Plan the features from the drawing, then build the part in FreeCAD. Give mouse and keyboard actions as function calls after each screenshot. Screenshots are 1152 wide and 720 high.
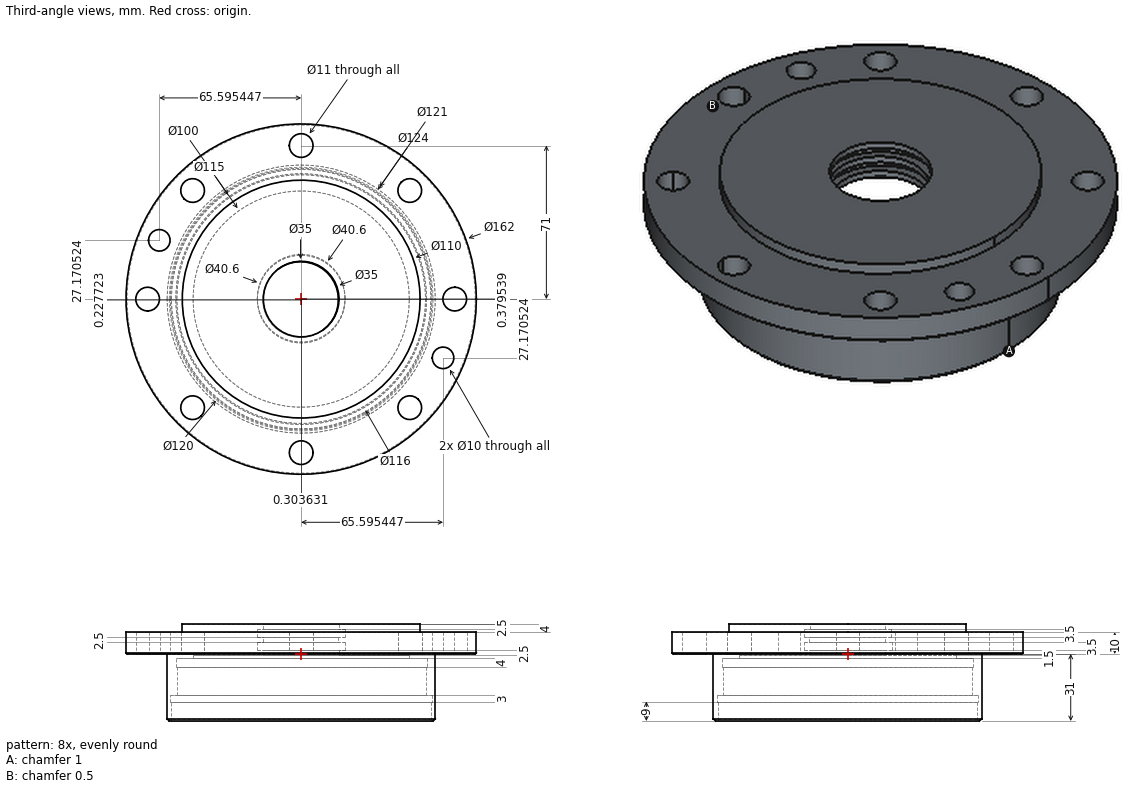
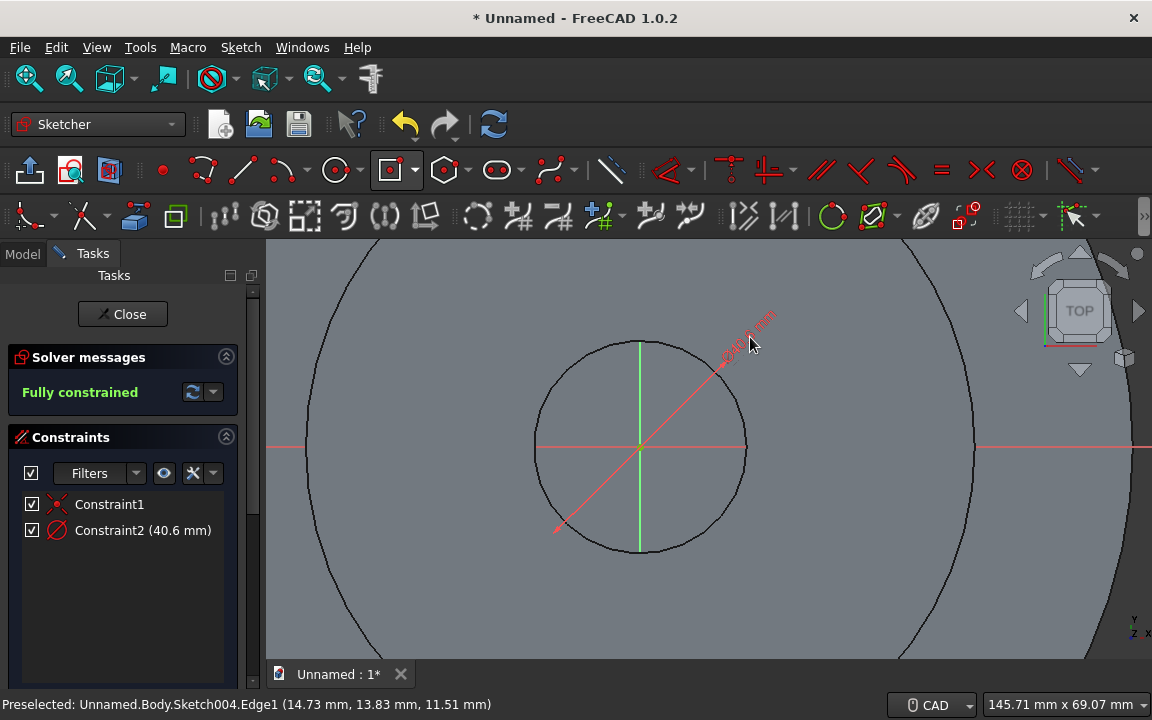
click(123, 314)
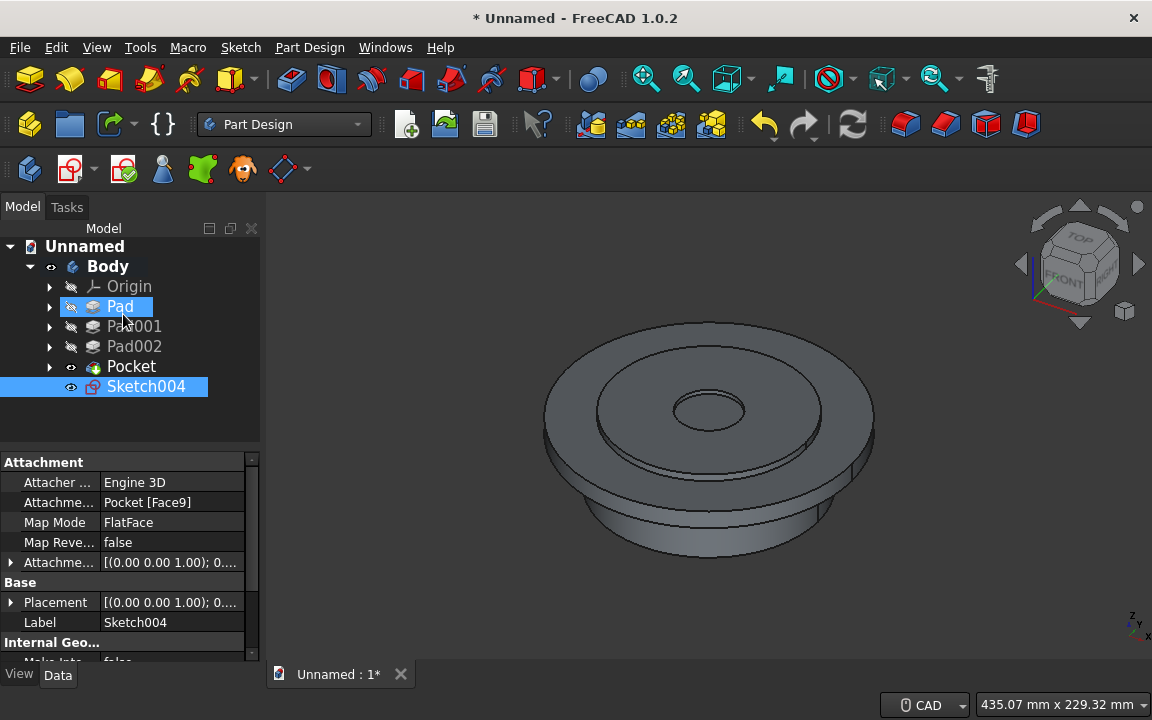
click(292, 80)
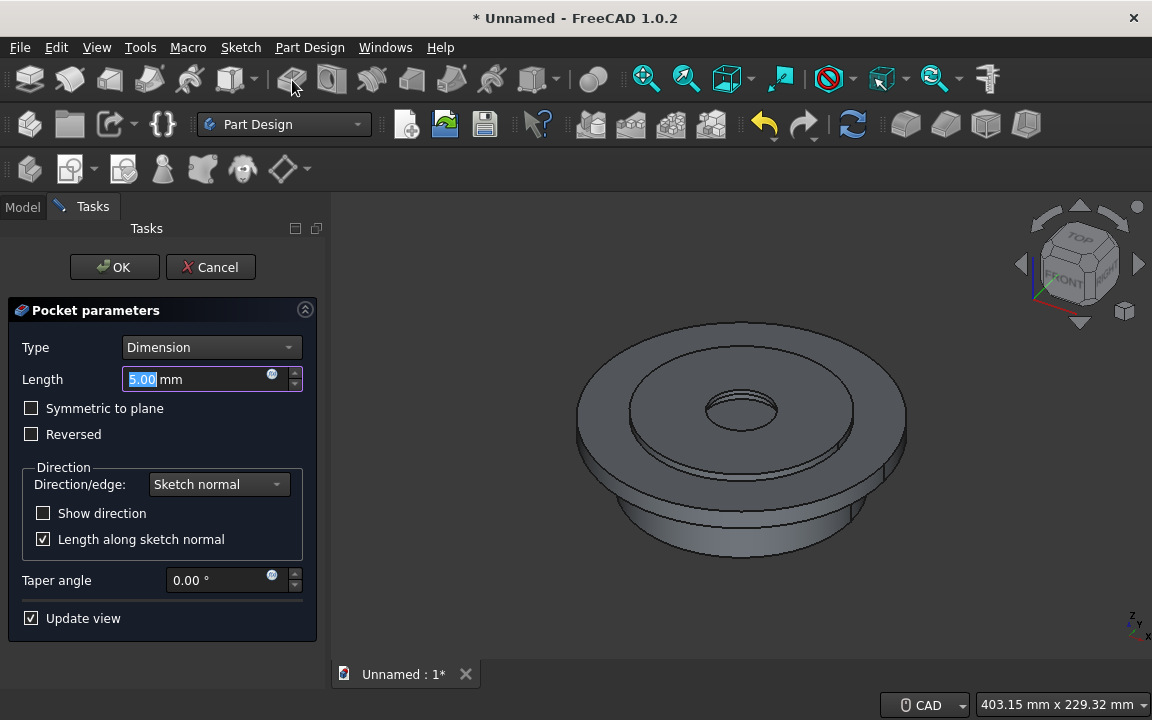
text(3.5)
key(Tab)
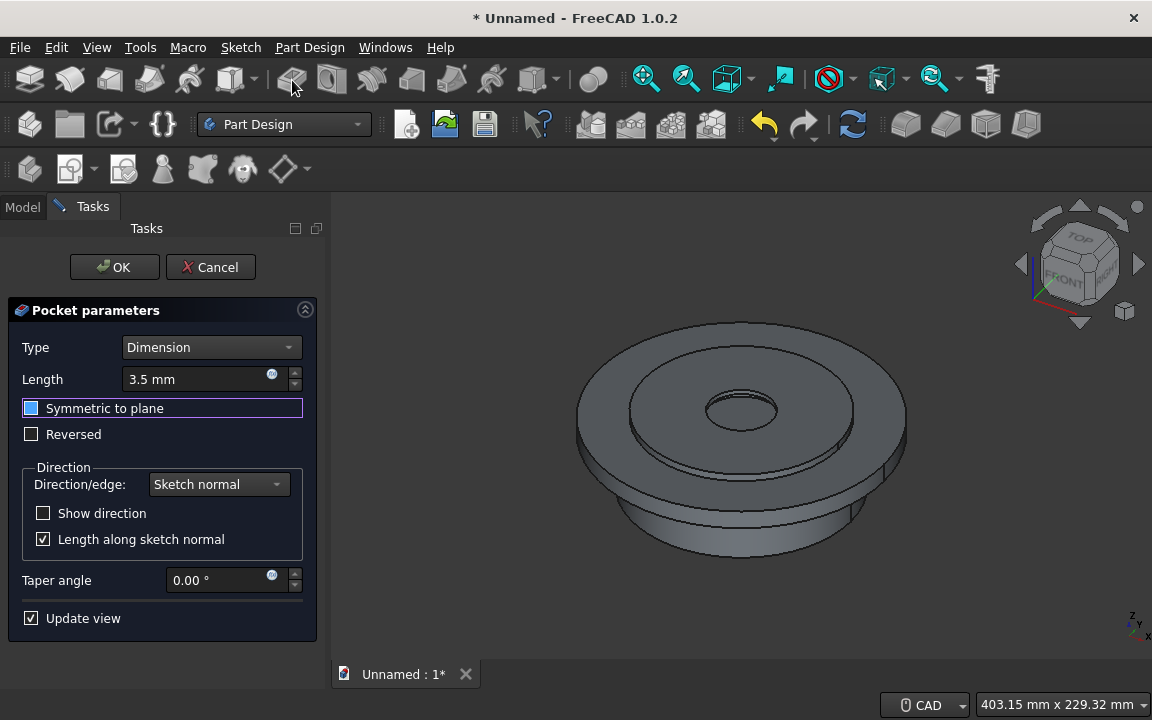
click(115, 267)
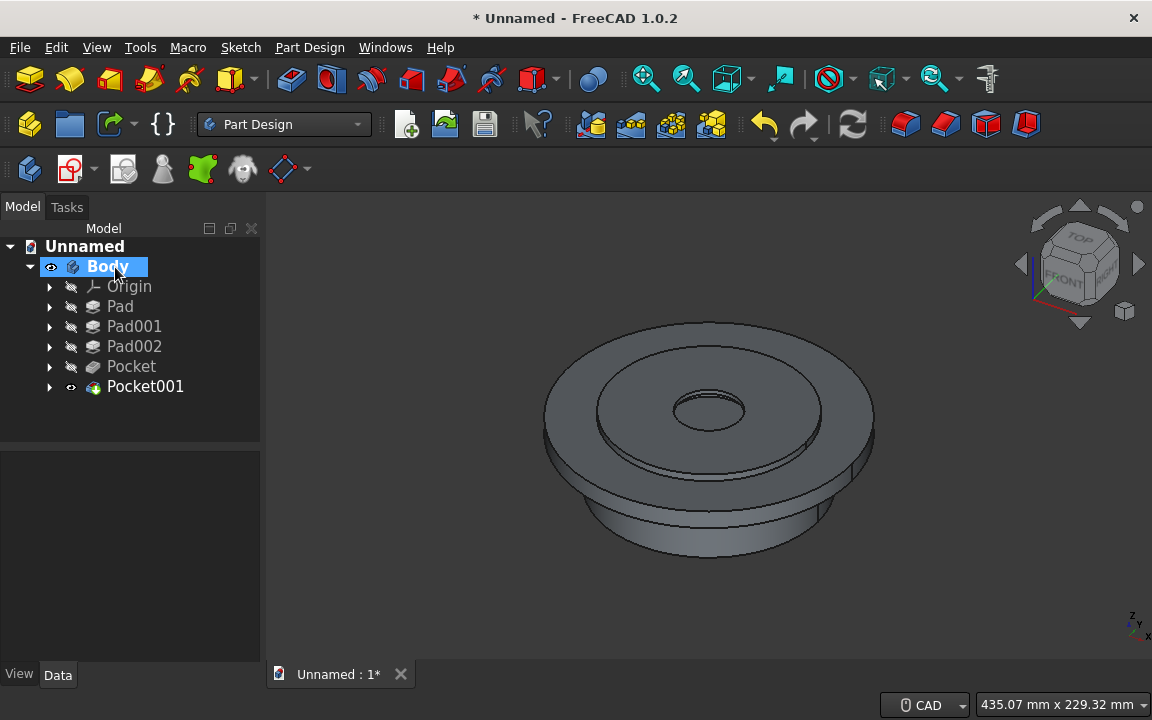
click(709, 419)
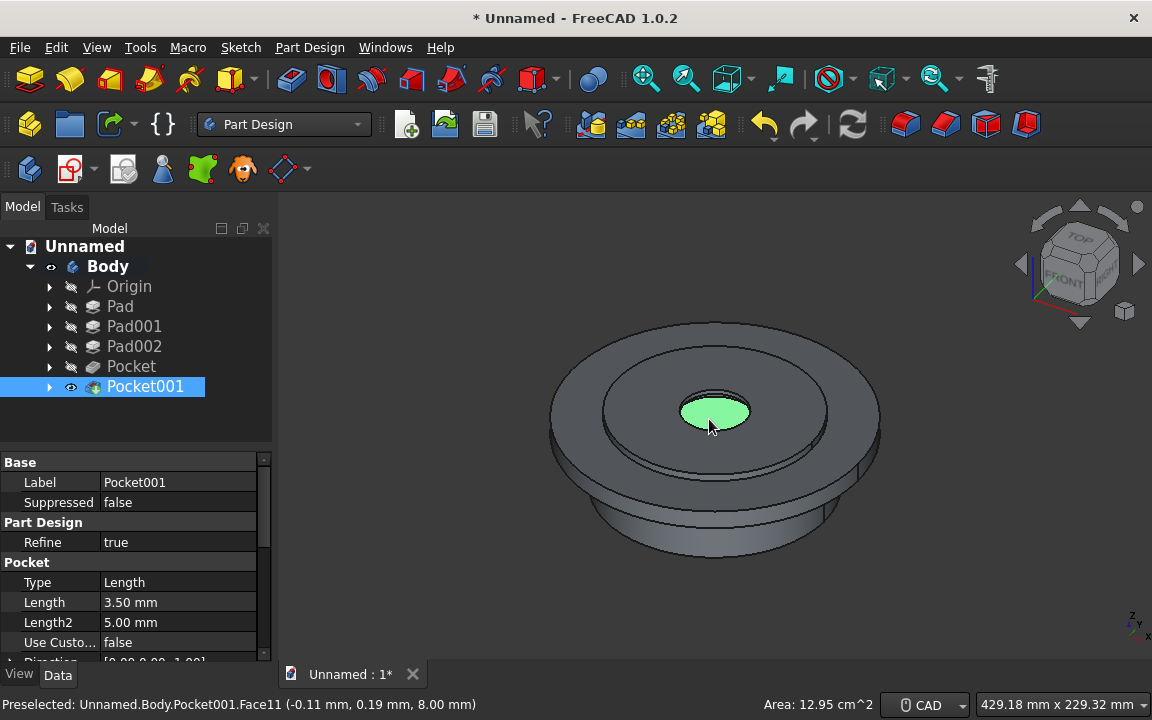
click(70, 170)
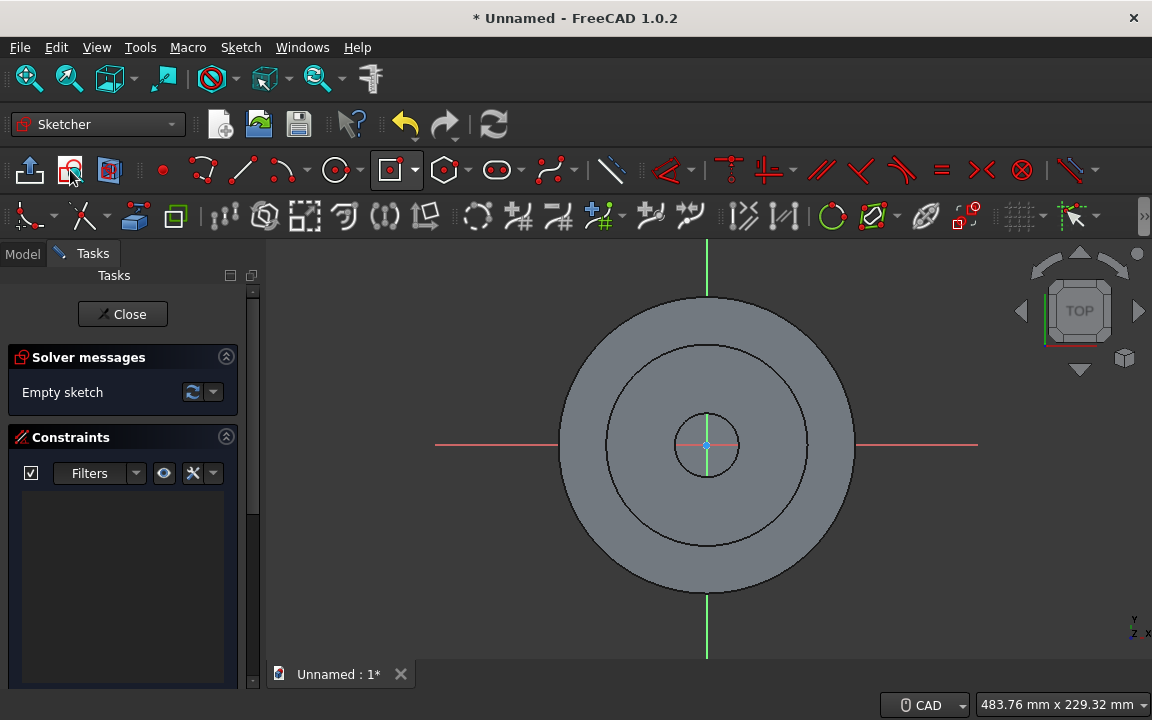
key(q)
key(s)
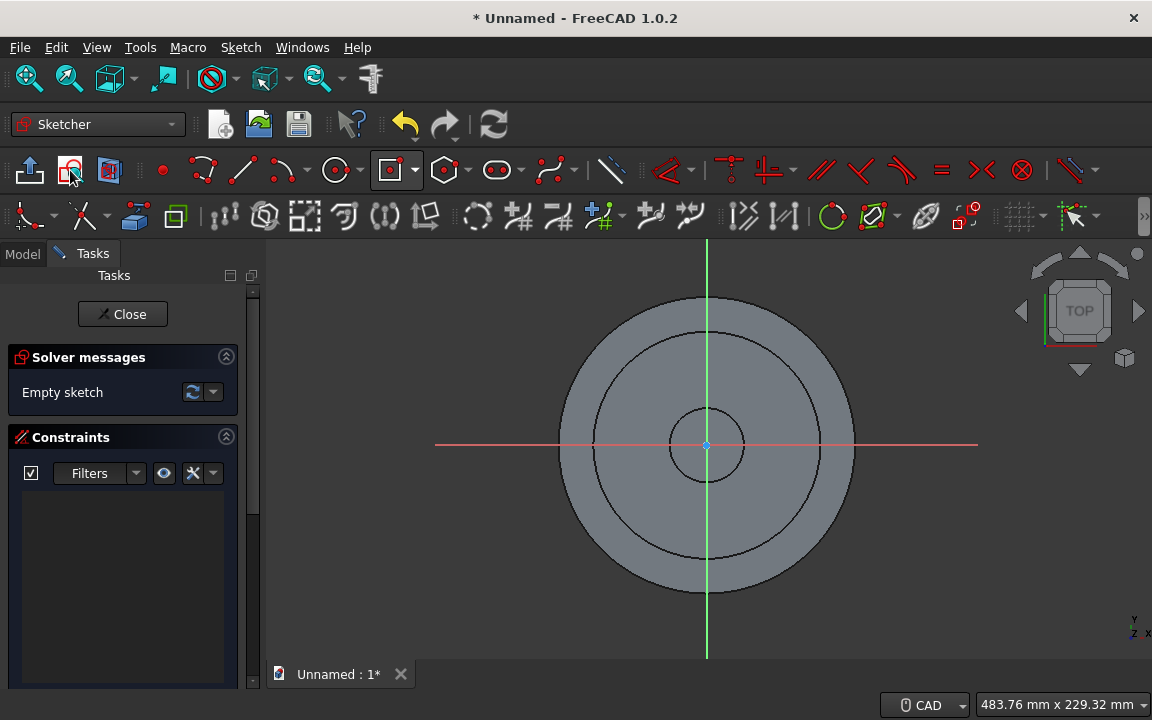
scroll(728, 445, up, 7)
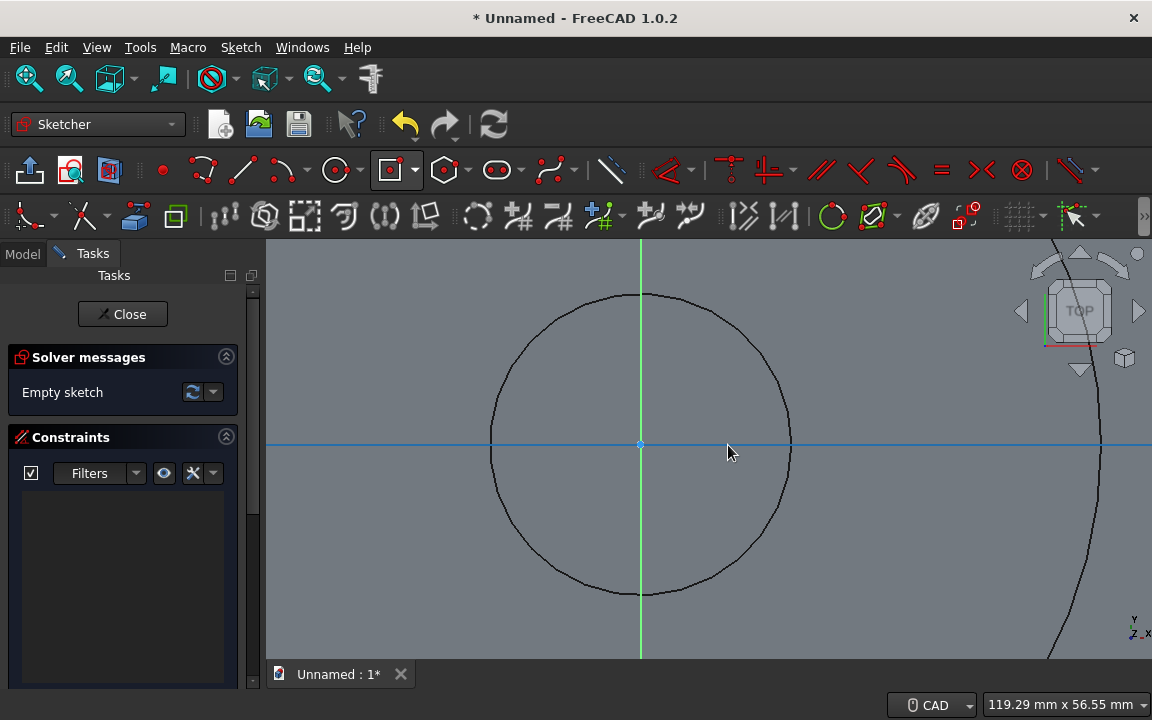
click(336, 170)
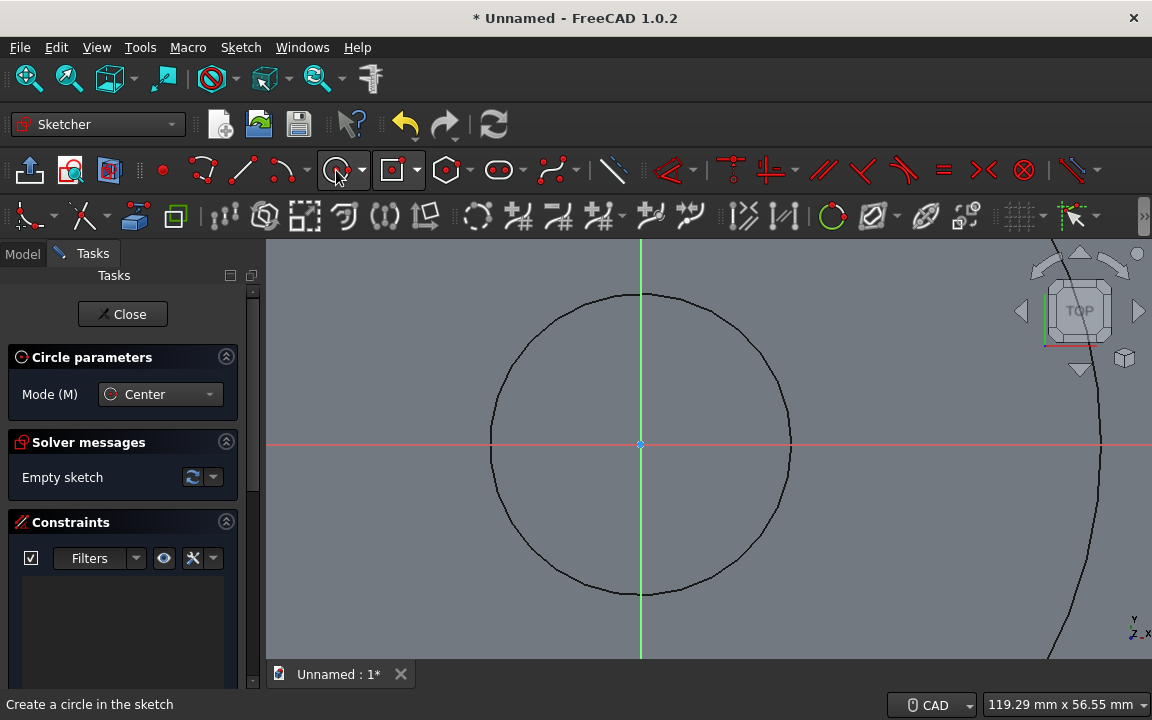
scroll(638, 446, up, 12)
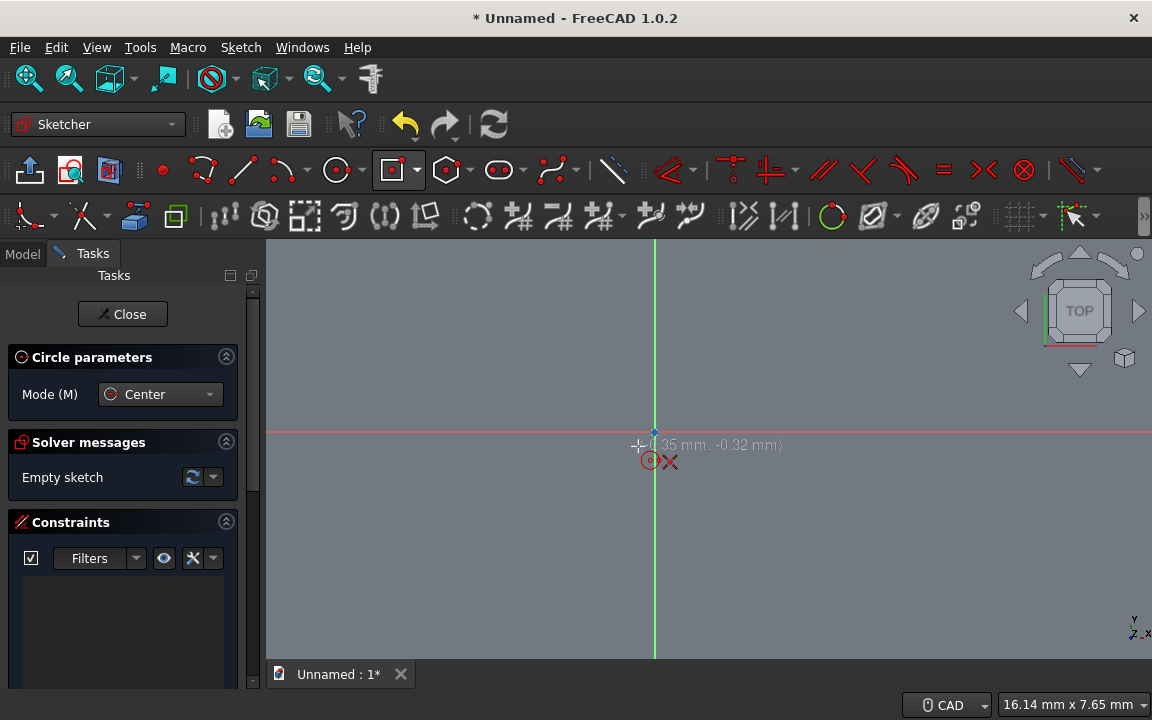
click(638, 444)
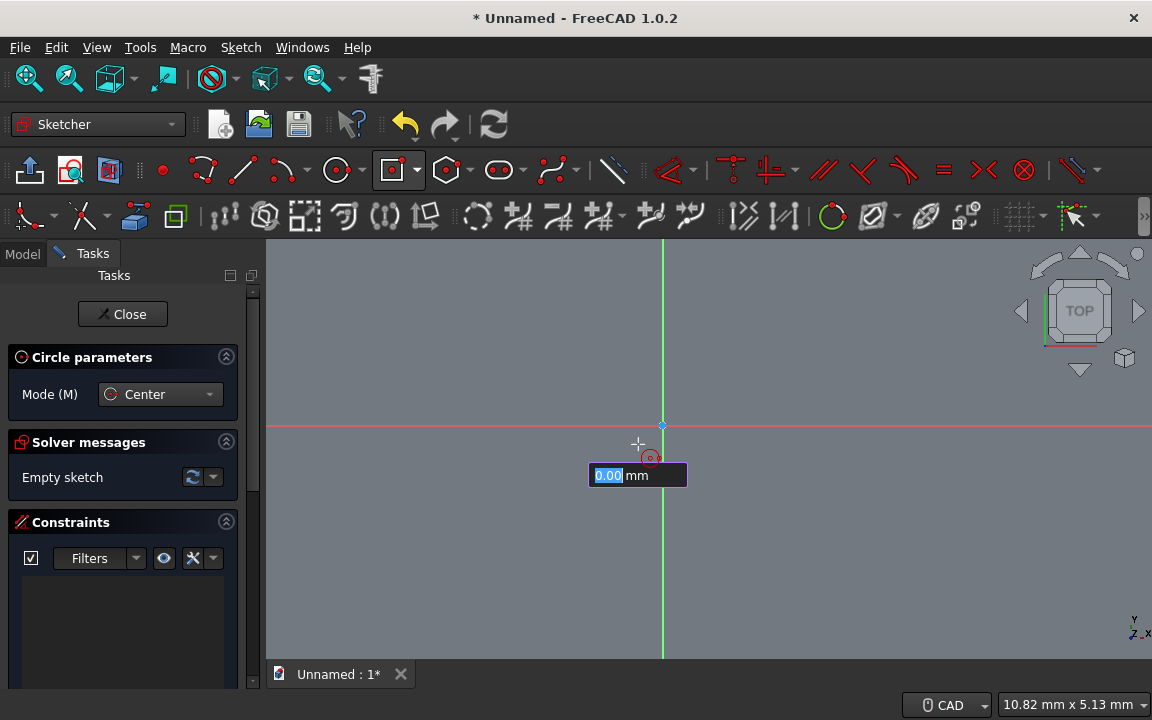
scroll(641, 449, down, 12)